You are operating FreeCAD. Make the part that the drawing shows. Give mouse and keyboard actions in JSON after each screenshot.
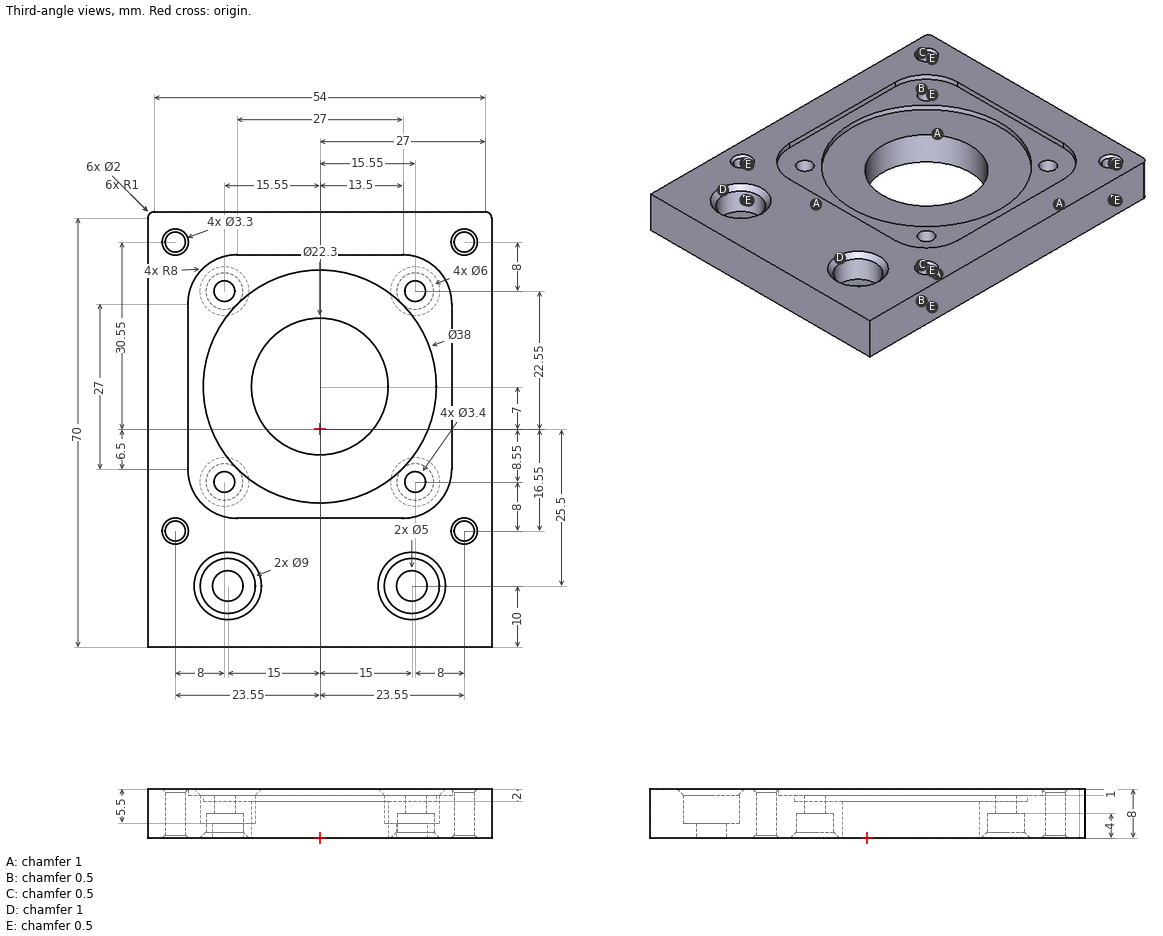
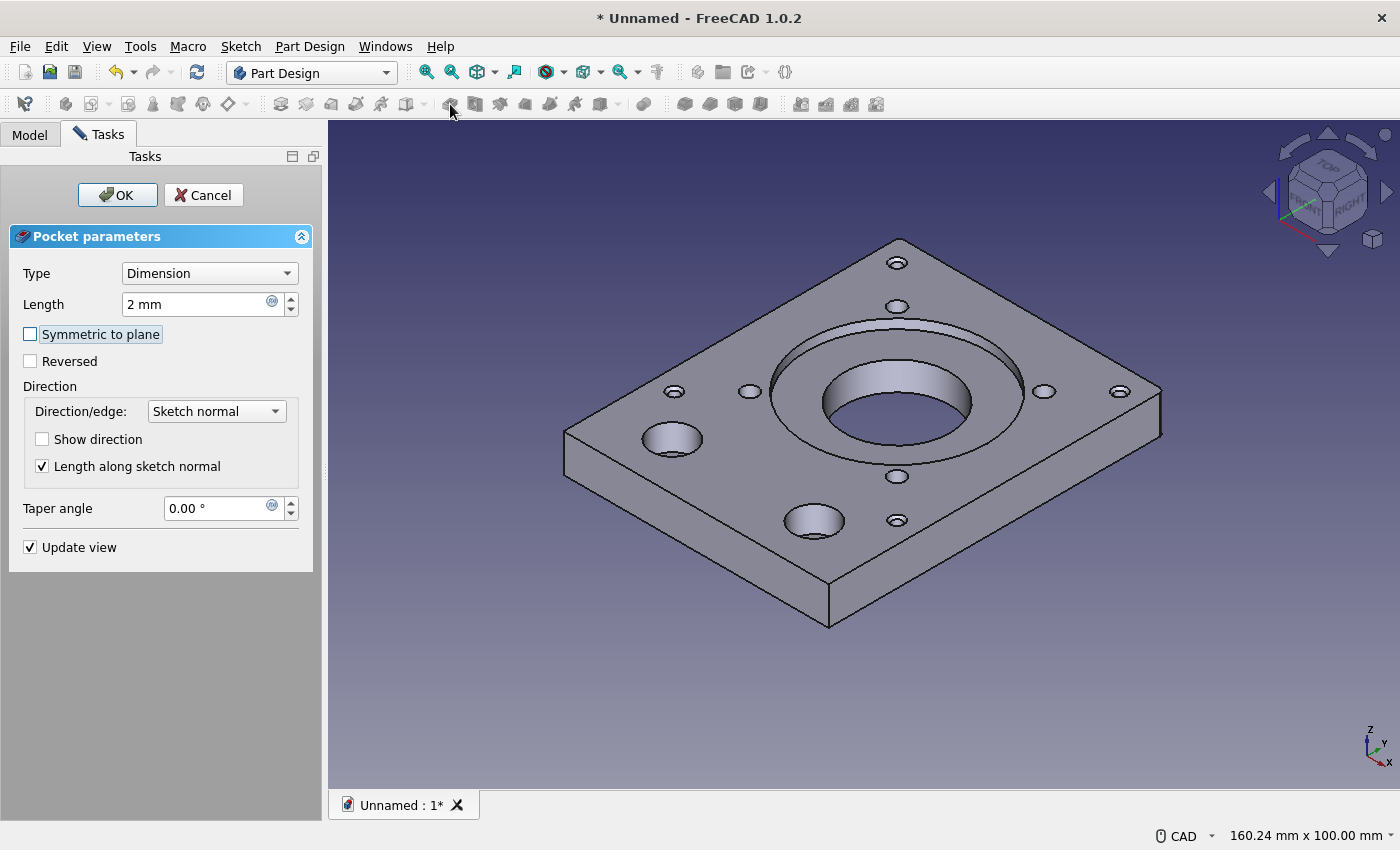
{"action": "left_click", "coordinate": [118, 195]}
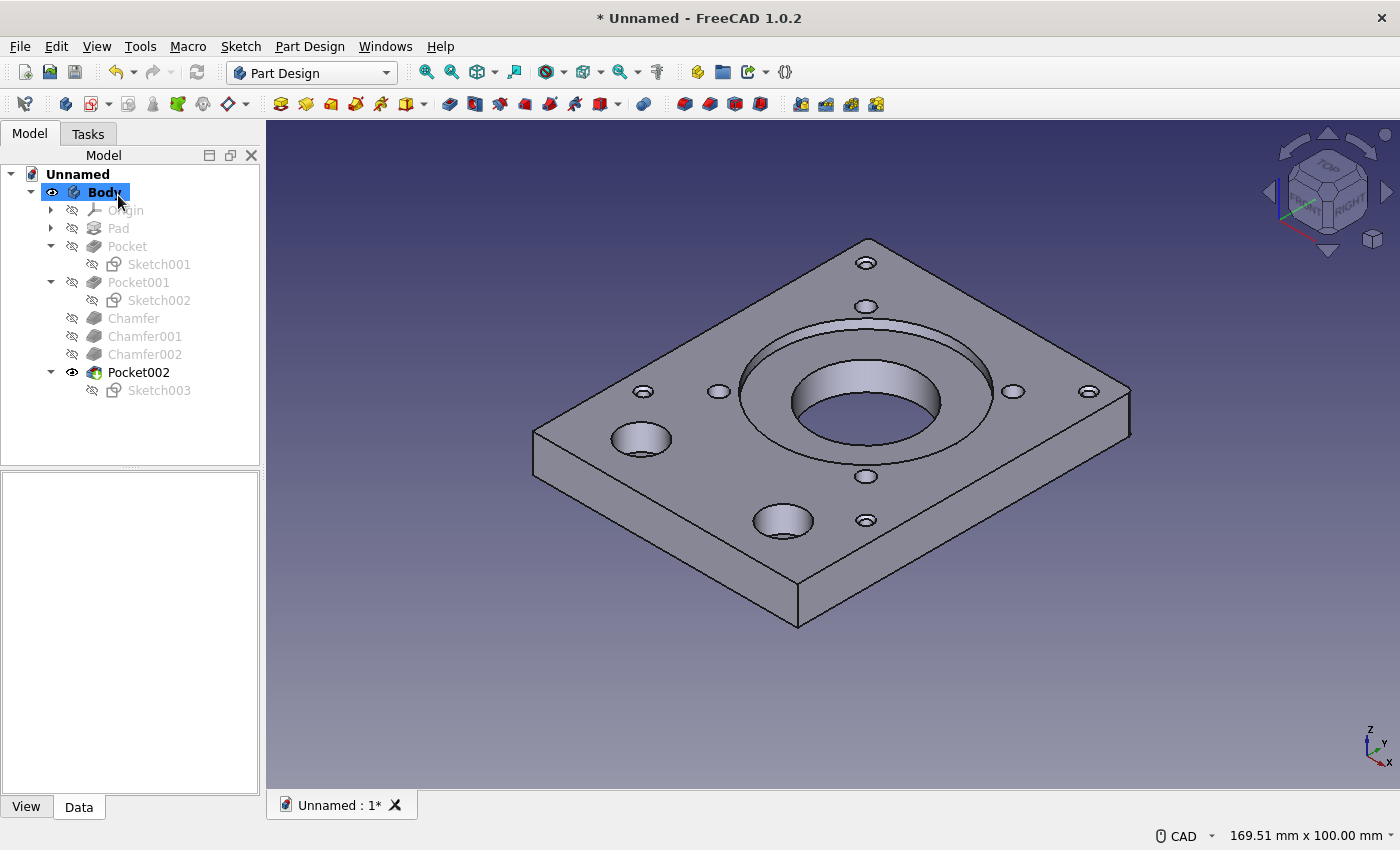
{"action": "left_click", "coordinate": [737, 465]}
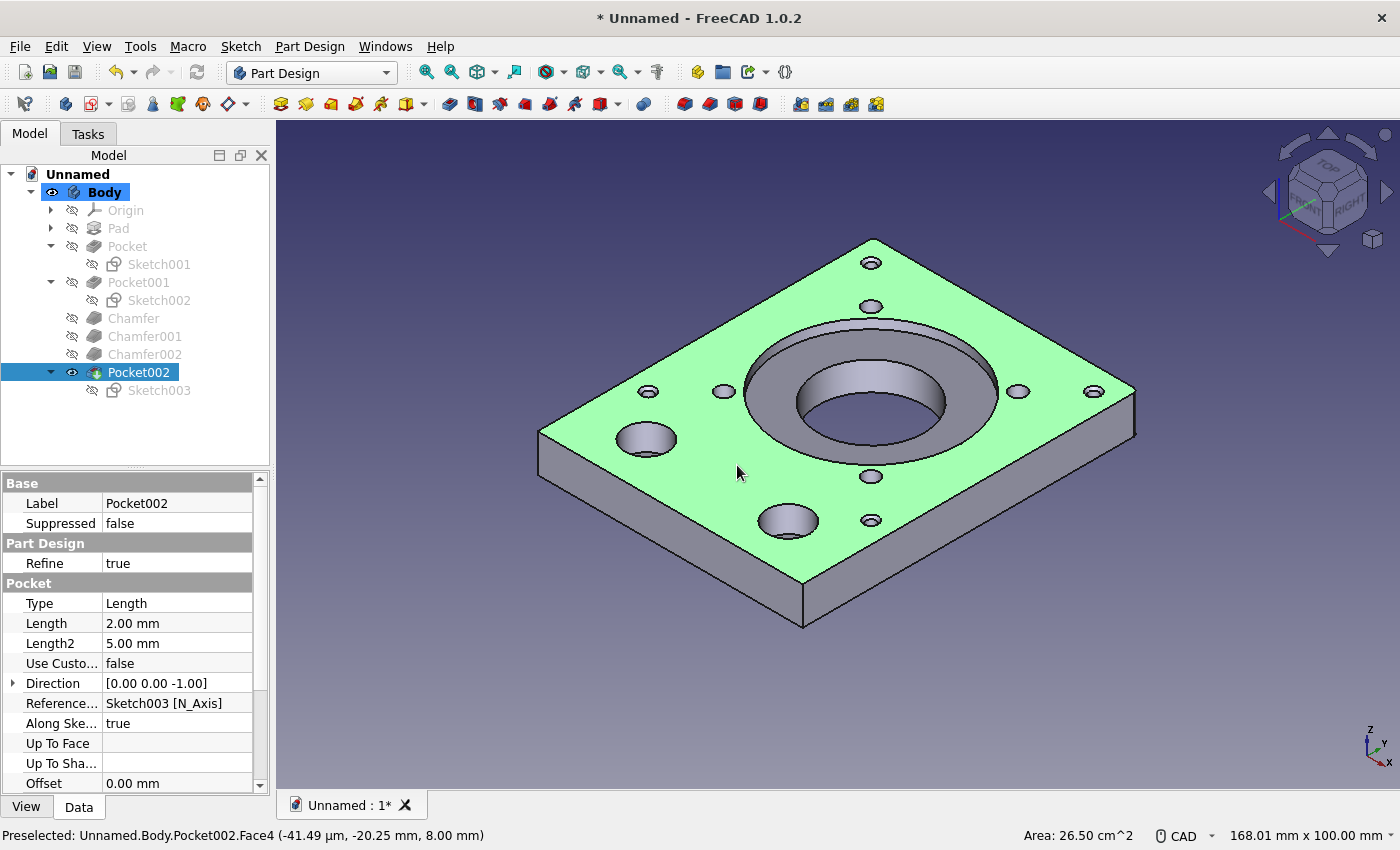
{"action": "left_click", "coordinate": [90, 104]}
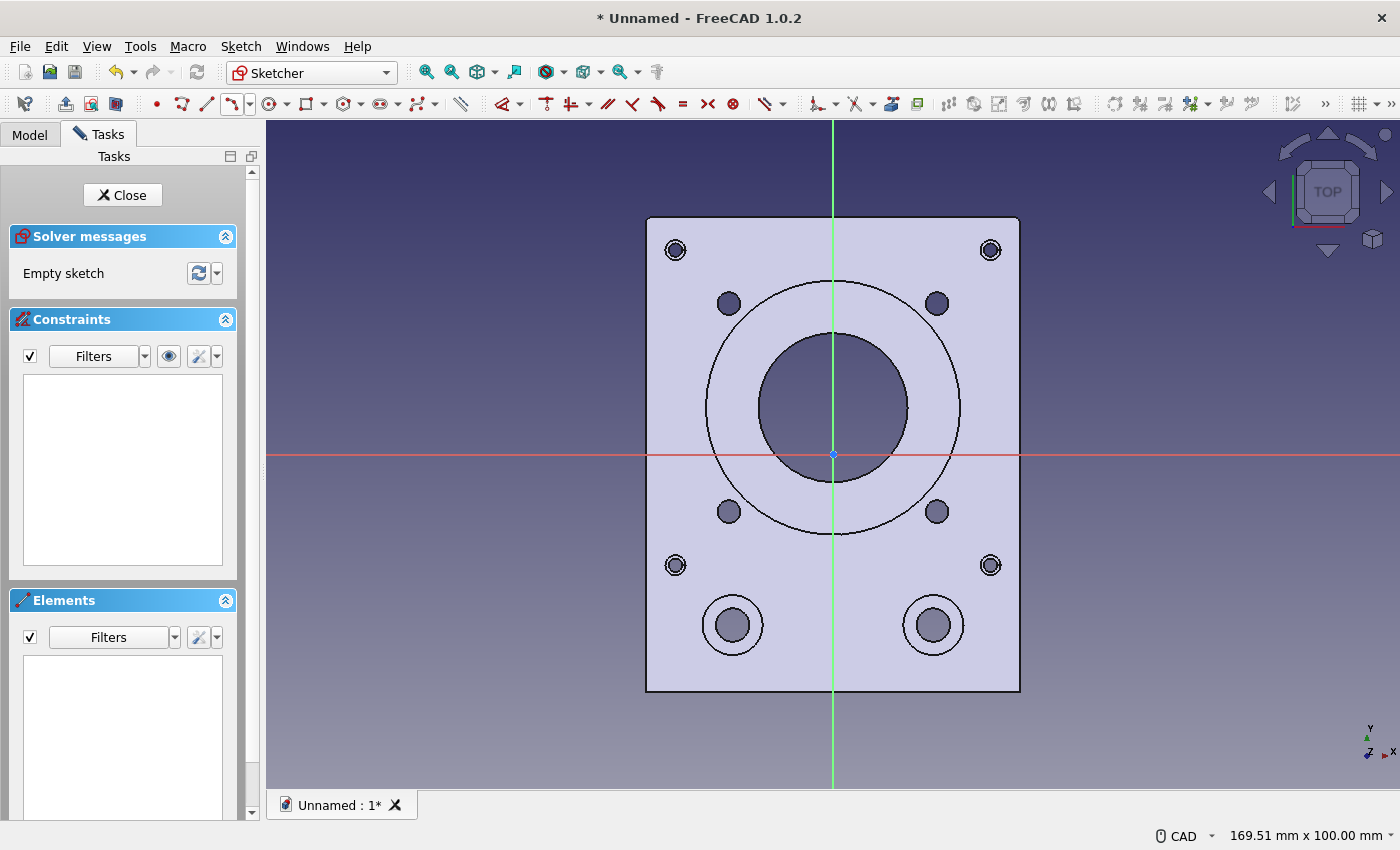
{"action": "scroll", "coordinate": [972, 312], "scroll_direction": "up", "scroll_amount": 2}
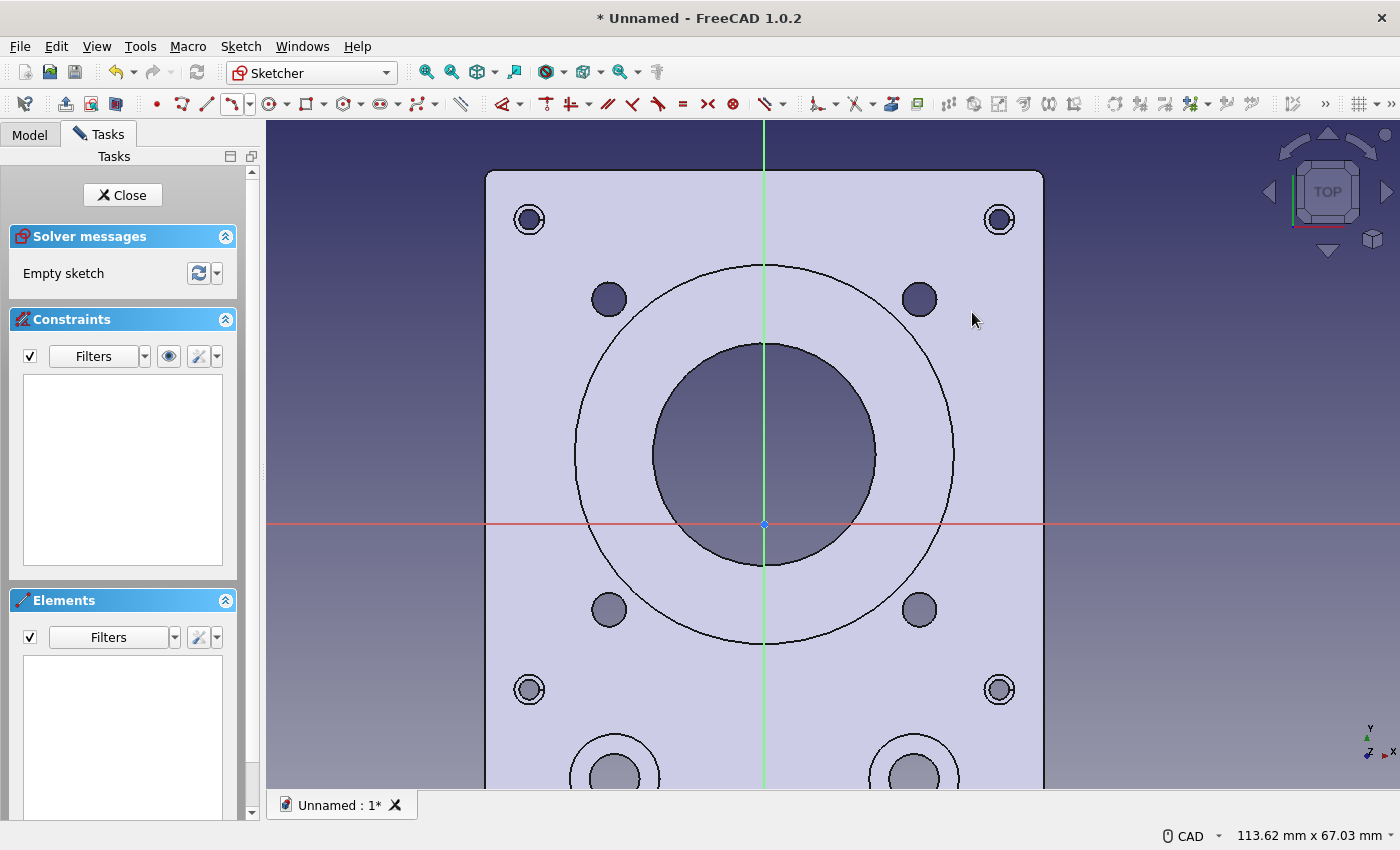
{"action": "key", "text": "g l"}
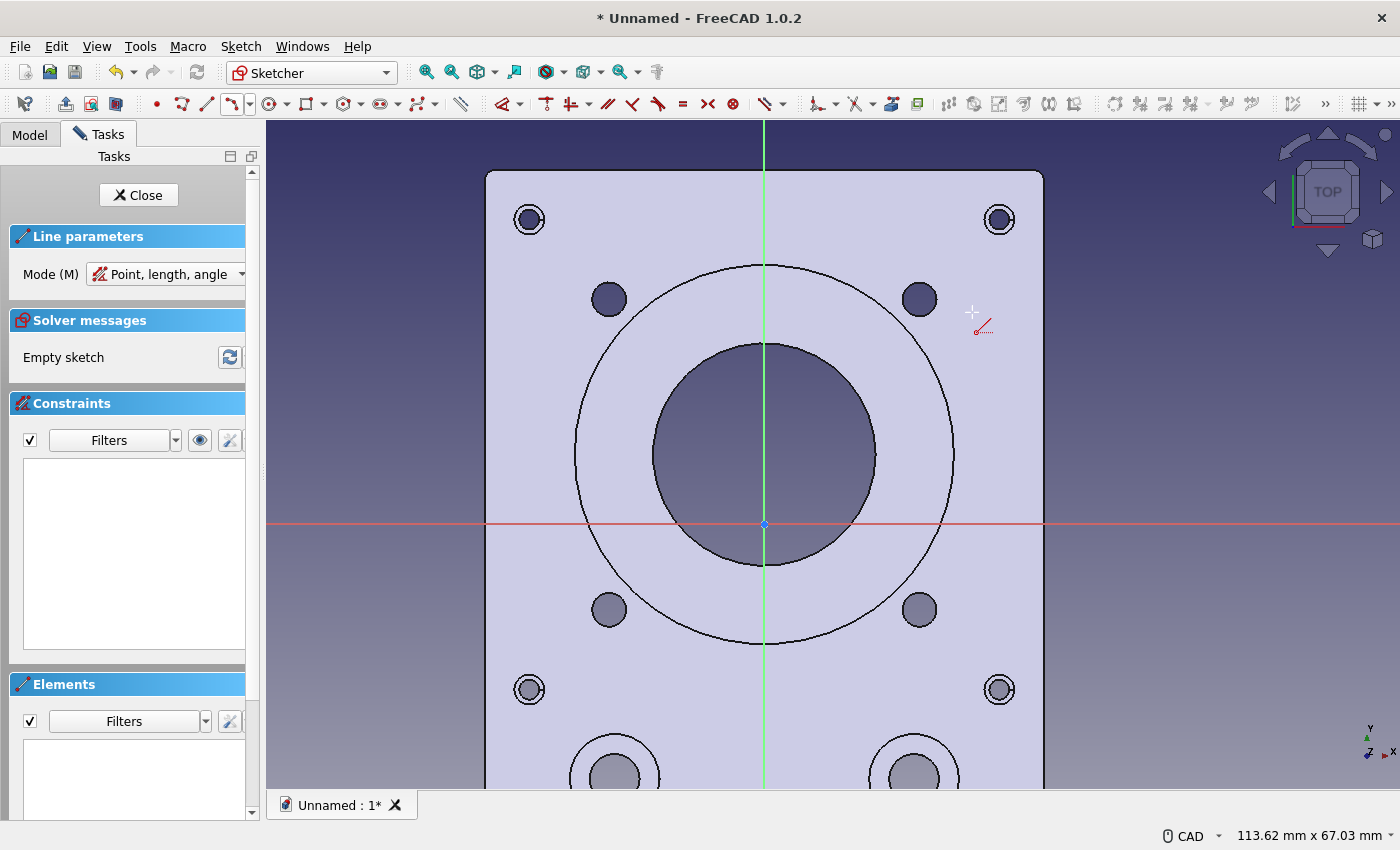
{"action": "left_click", "coordinate": [899, 240]}
{"action": "left_click", "coordinate": [630, 240]}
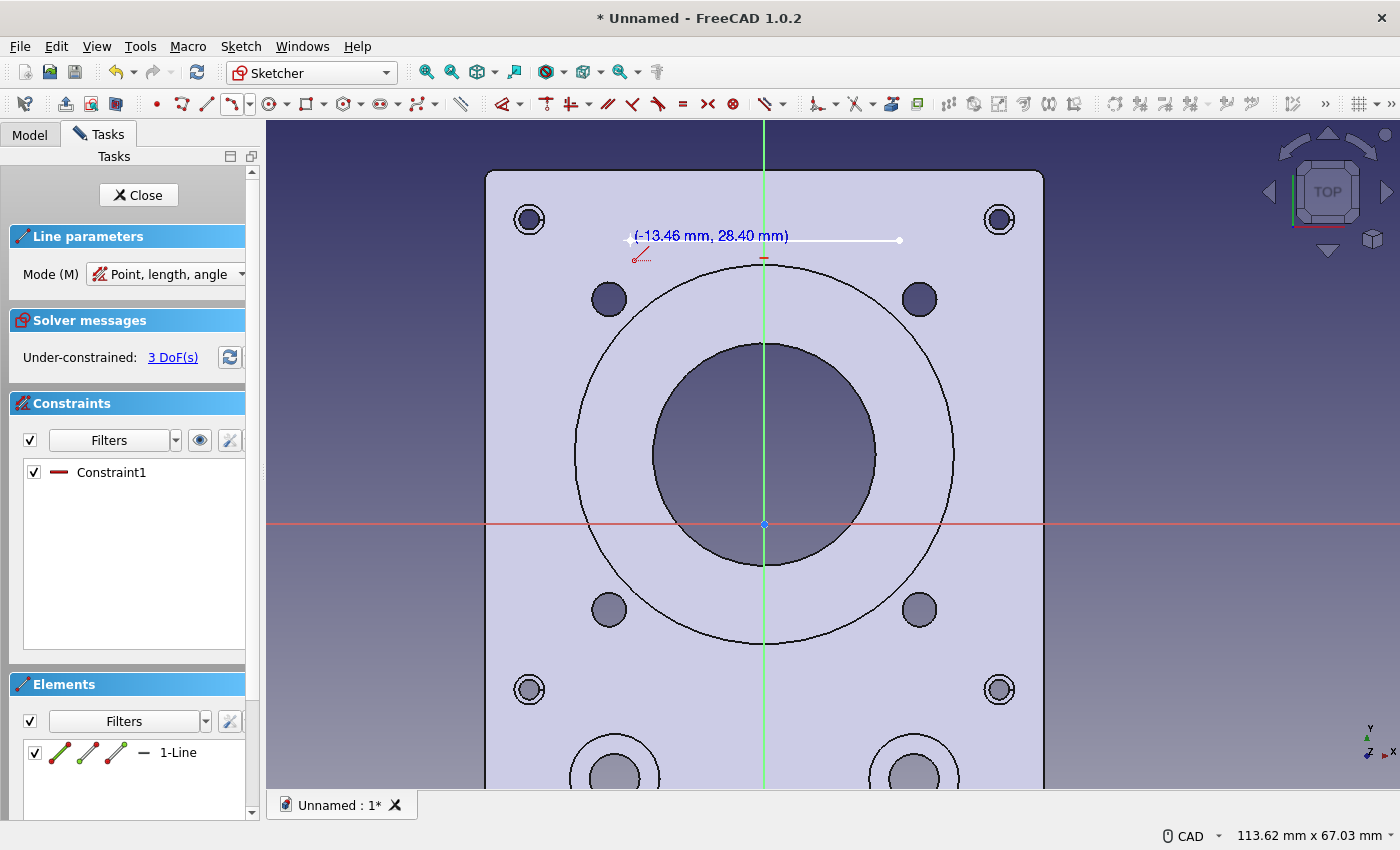
{"action": "left_click", "coordinate": [550, 320]}
{"action": "left_click", "coordinate": [550, 589]}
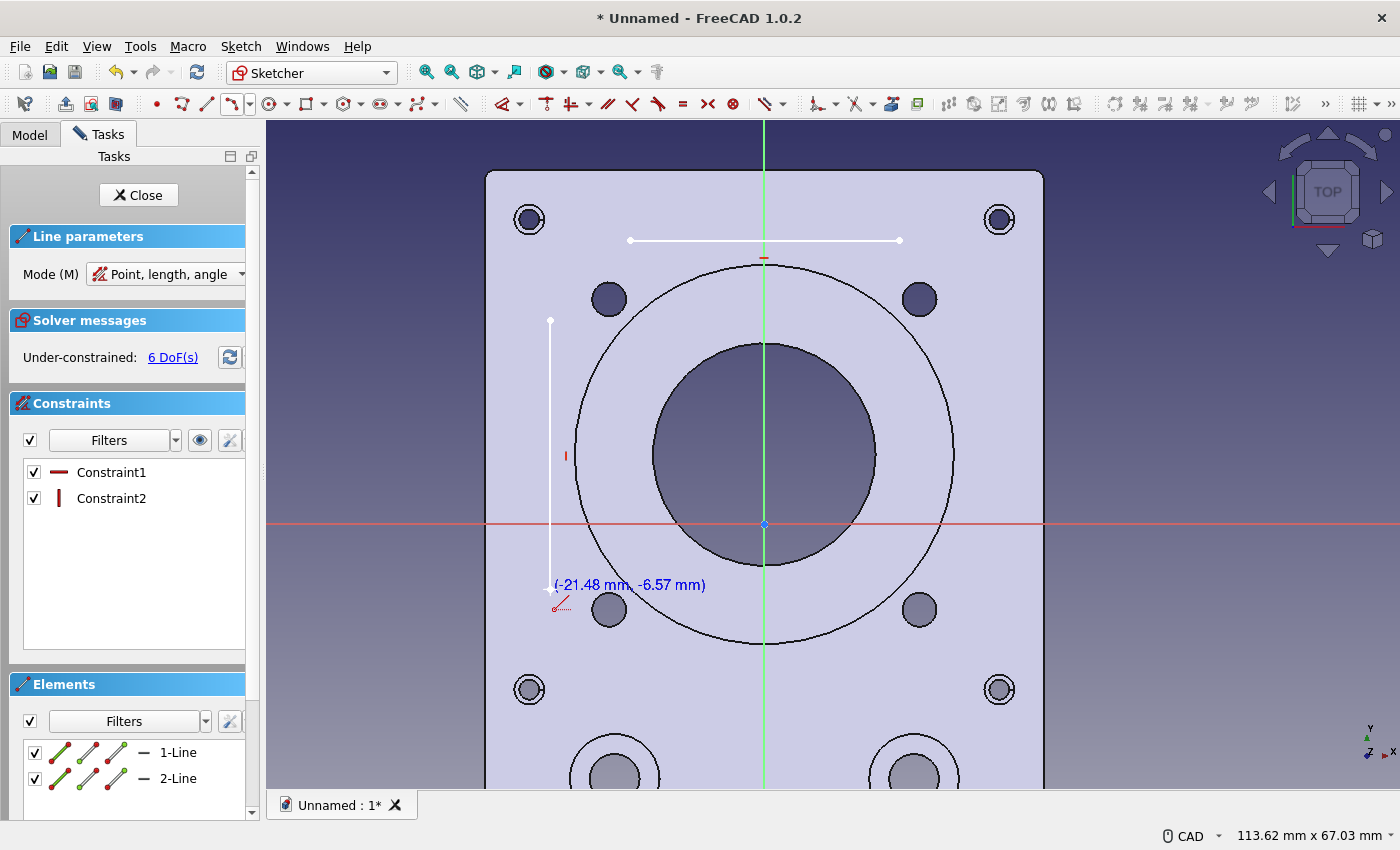
{"action": "left_click", "coordinate": [630, 669]}
{"action": "left_click", "coordinate": [899, 669]}